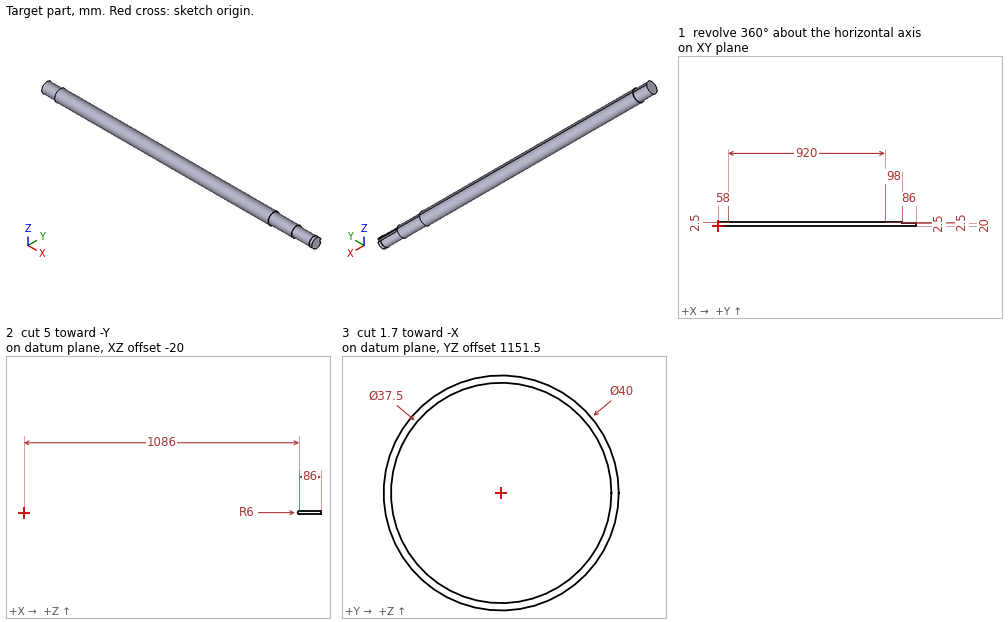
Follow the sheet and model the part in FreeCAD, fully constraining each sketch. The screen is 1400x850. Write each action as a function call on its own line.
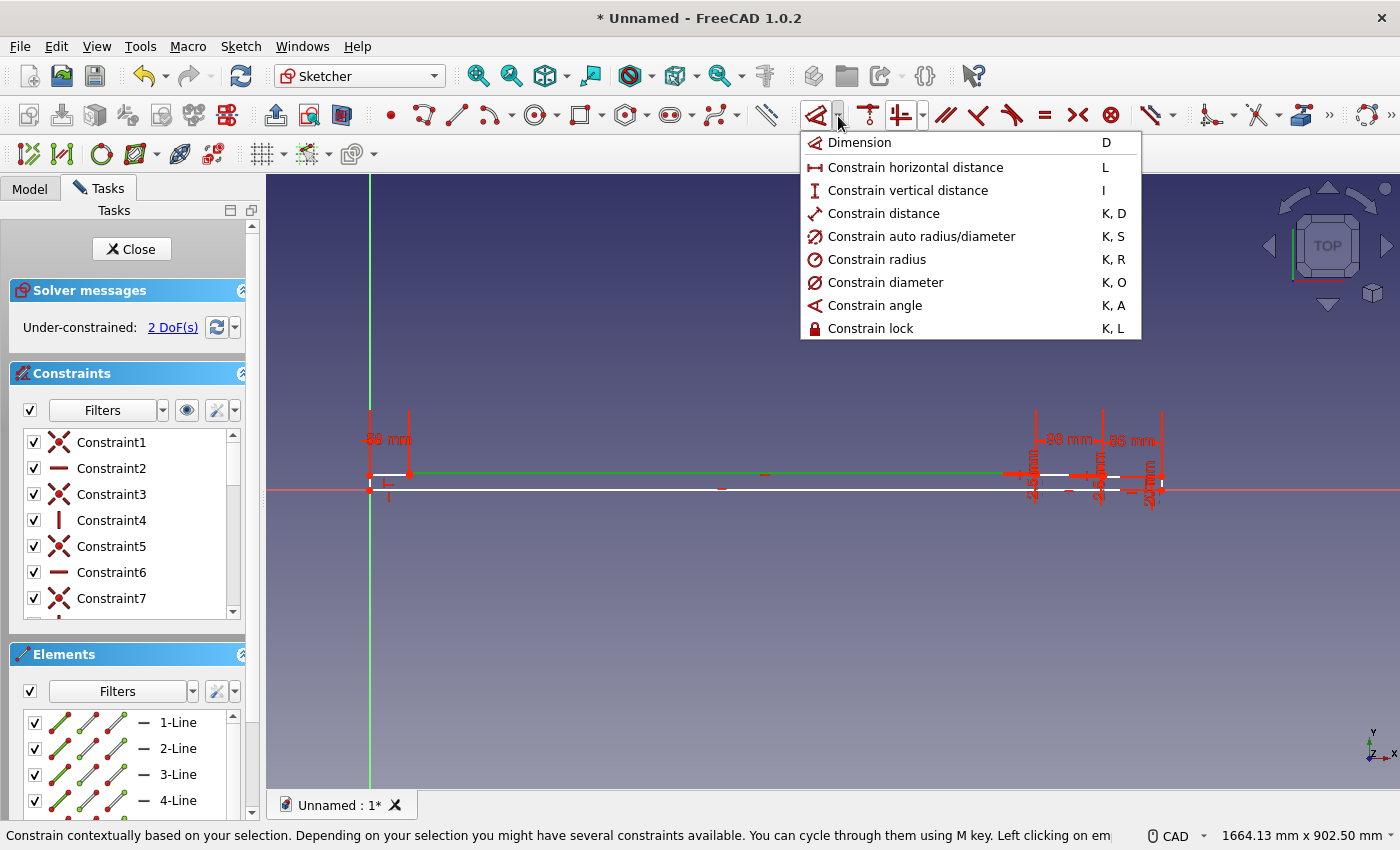
click(971, 168)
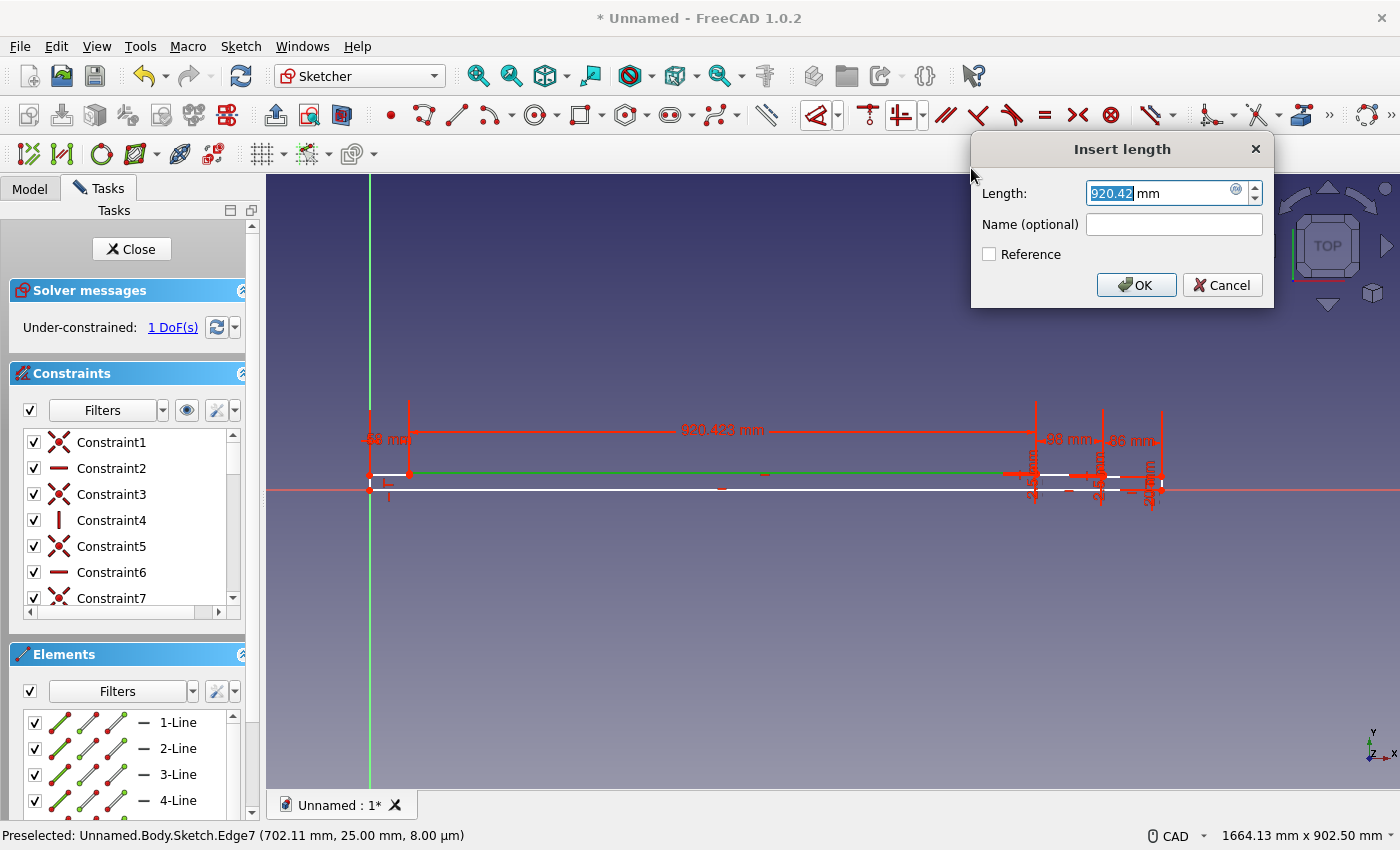
text(920)
key(Return)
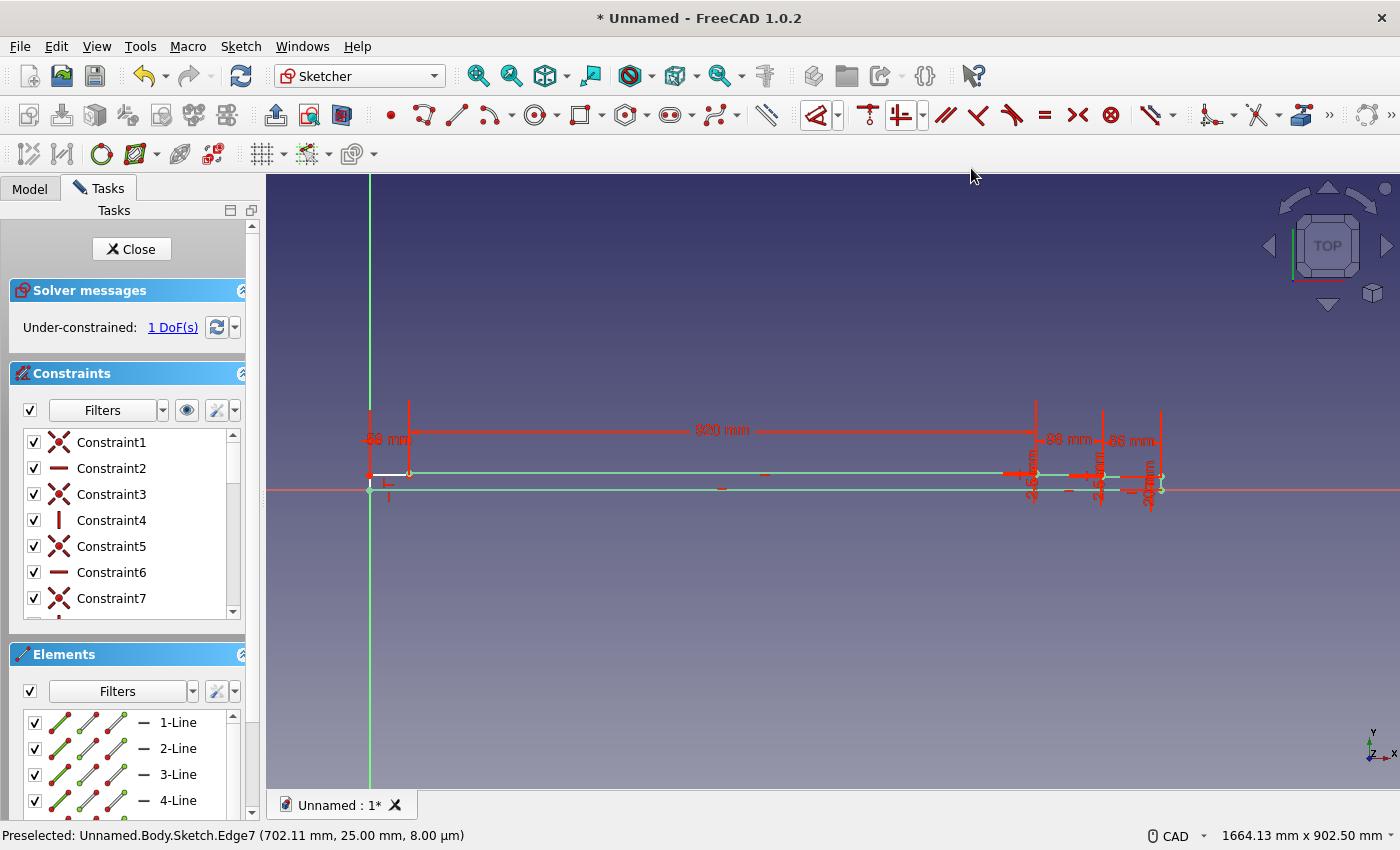
scroll(409, 474, up, 16)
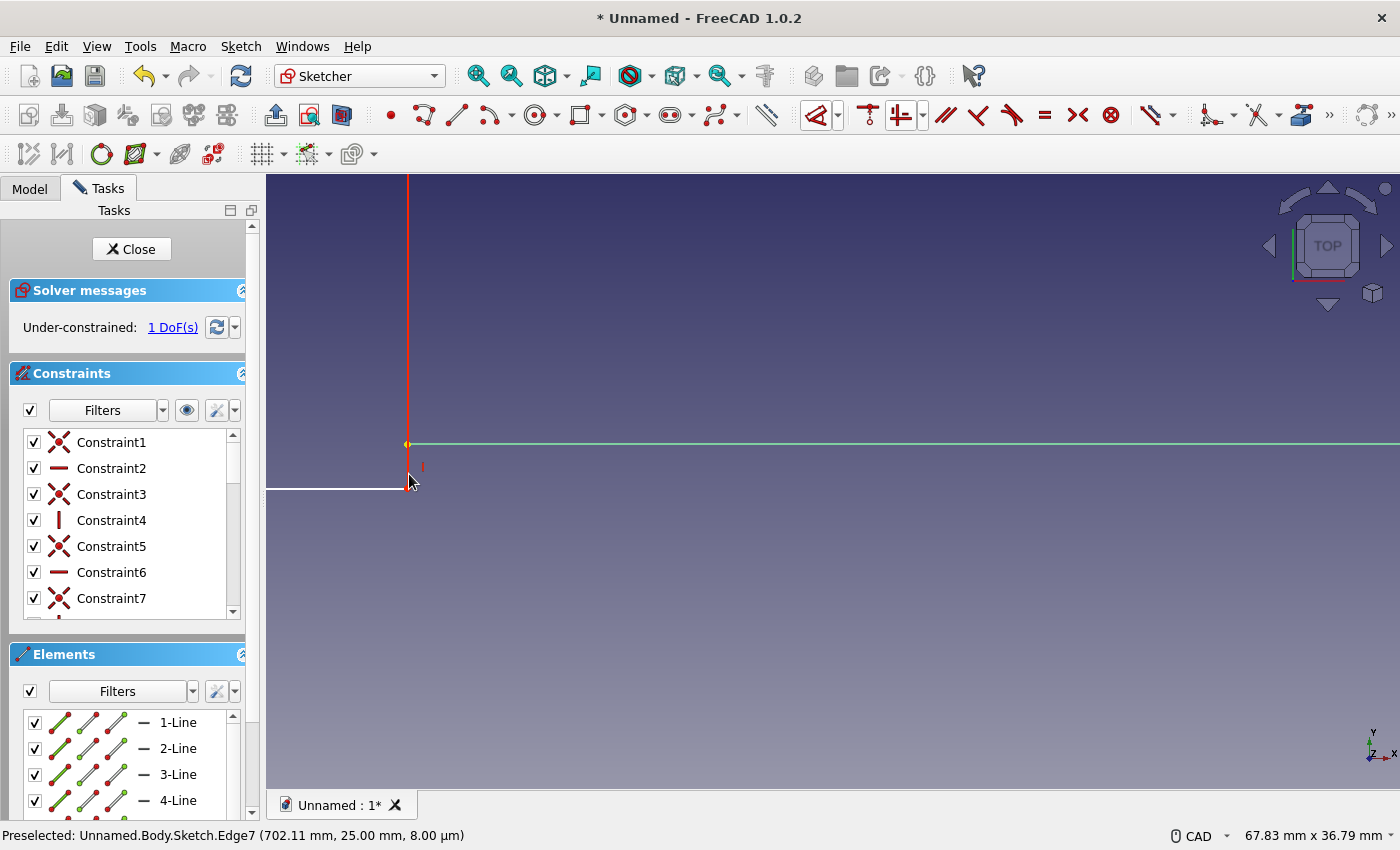
click(408, 466)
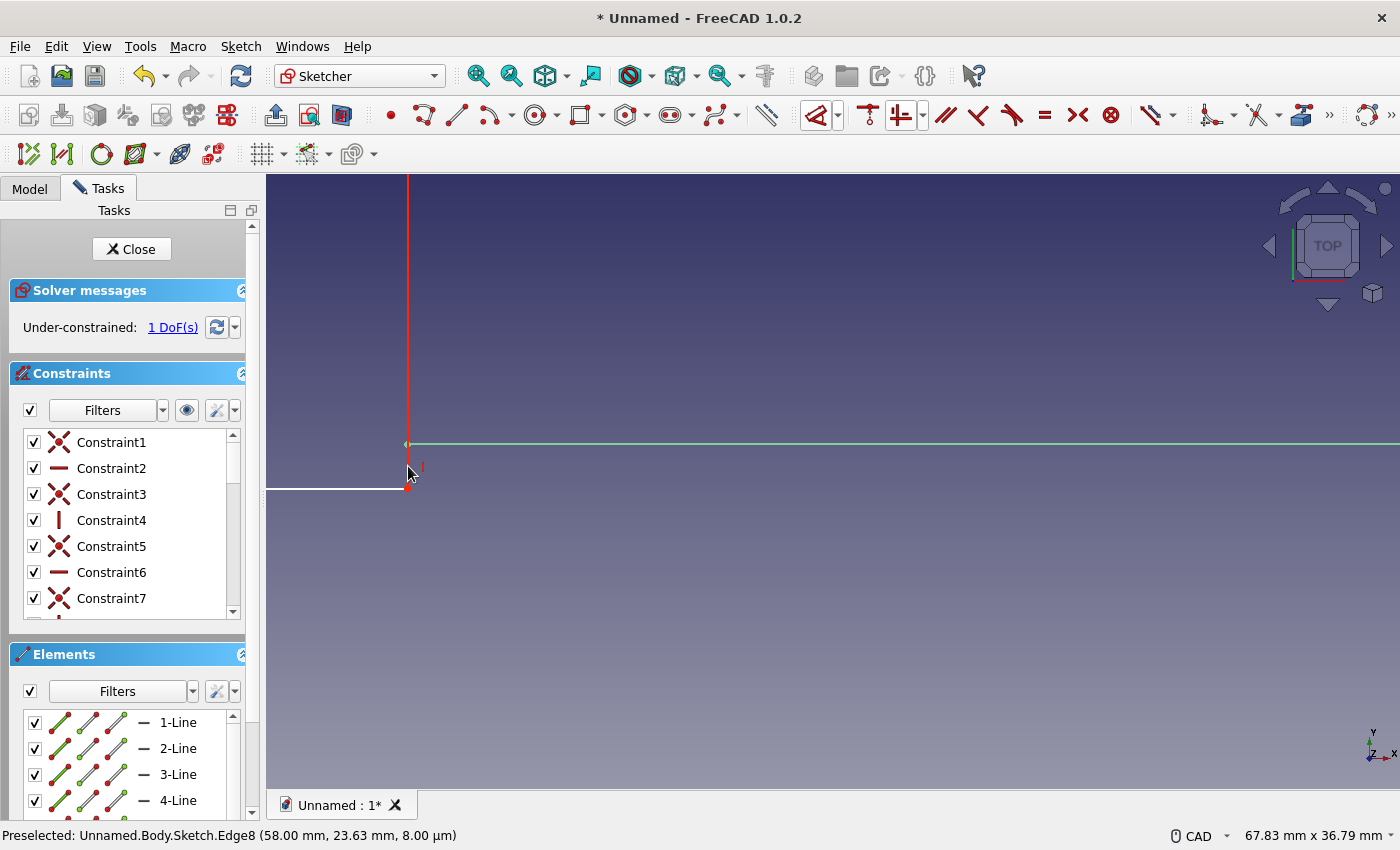
click(838, 116)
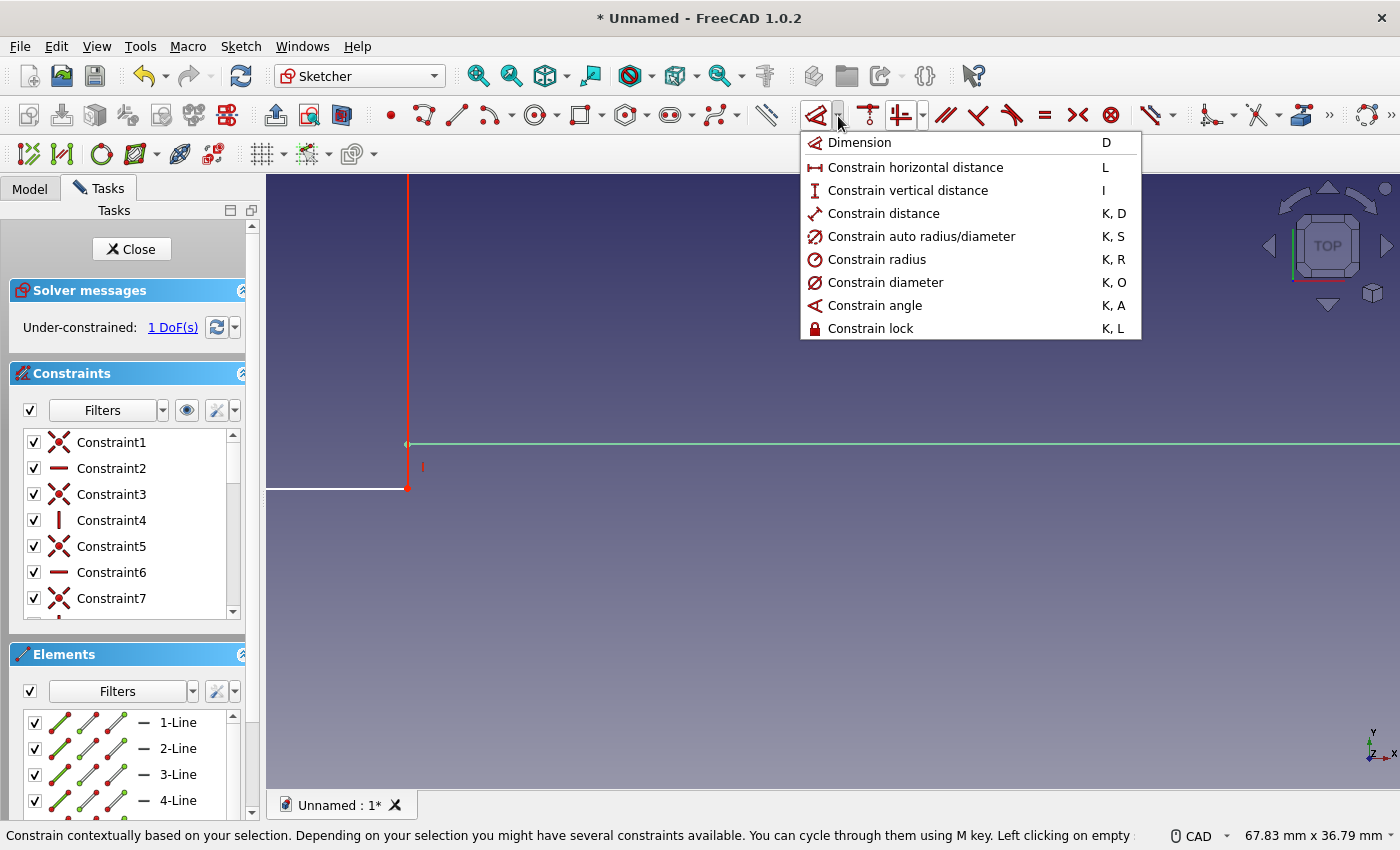
click(971, 190)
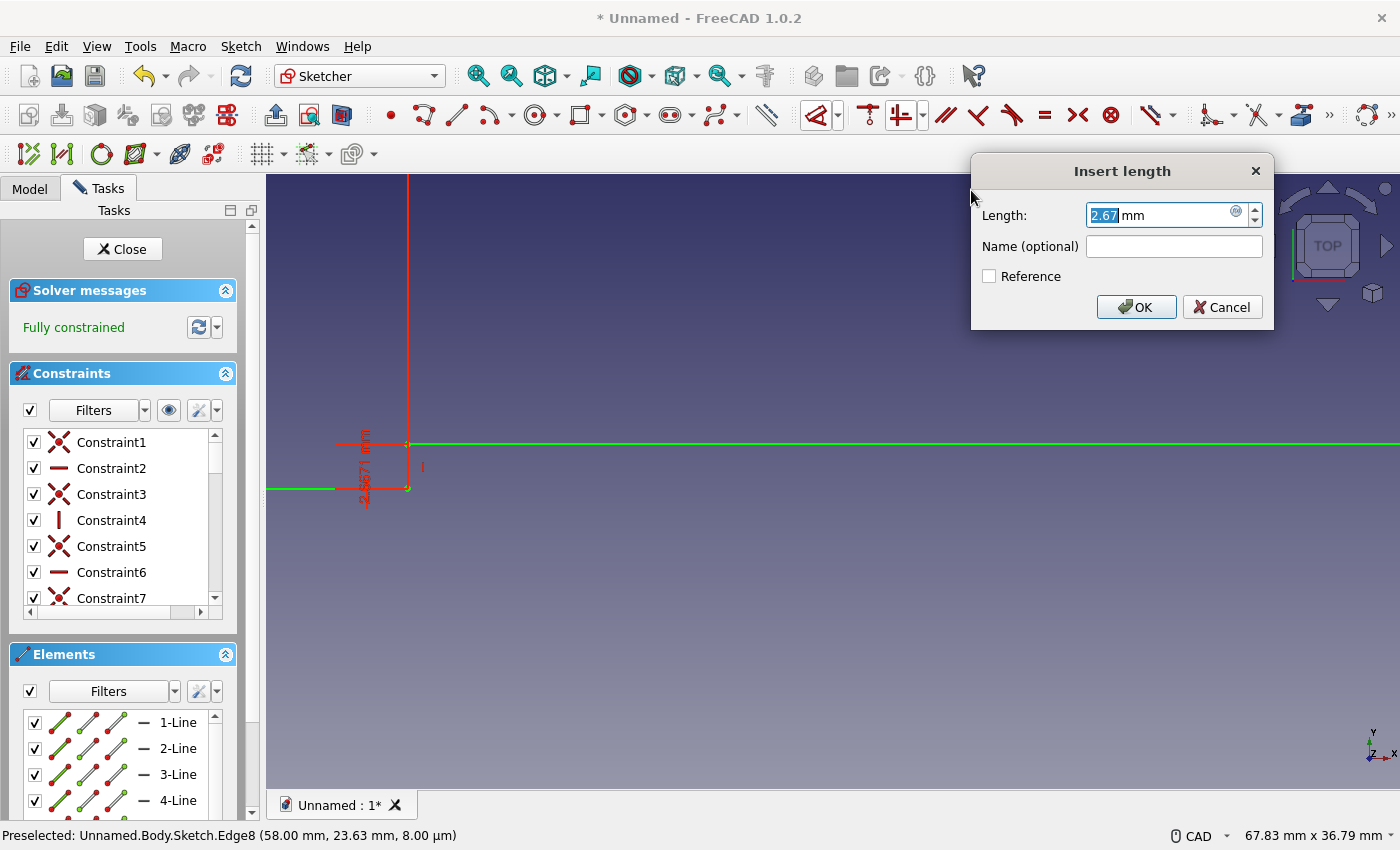
text(2.5)
key(Return)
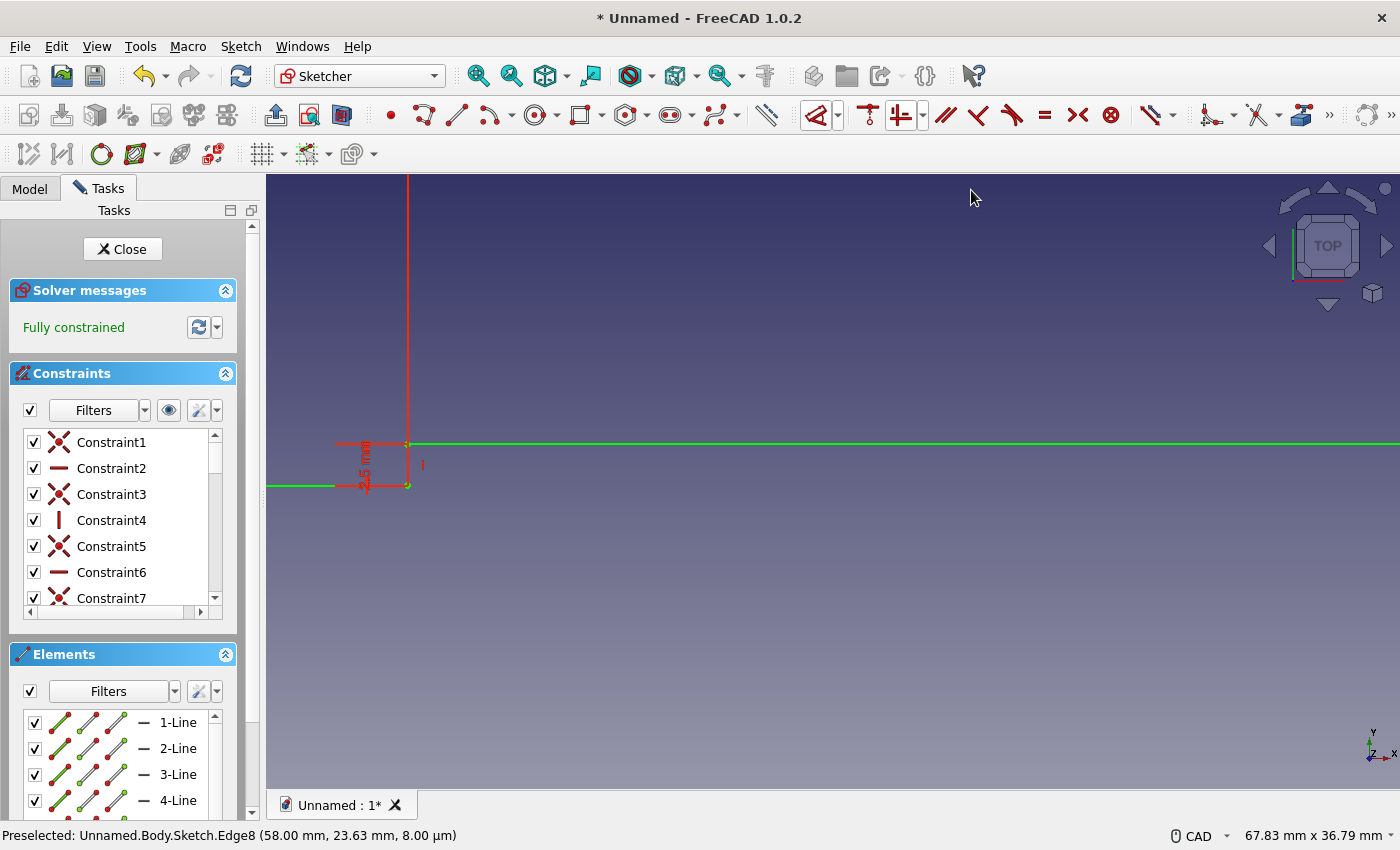
click(123, 249)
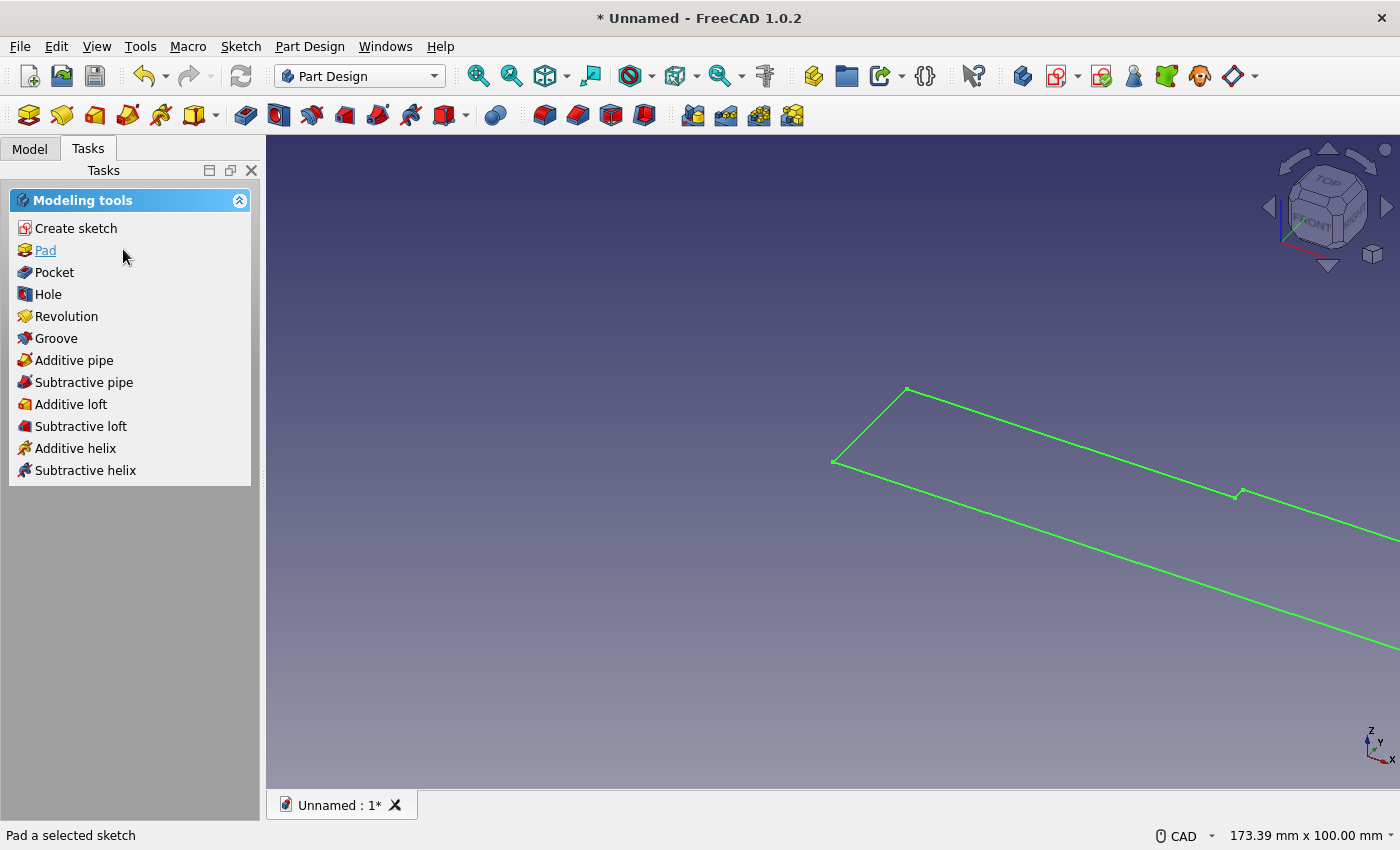
click(62, 116)